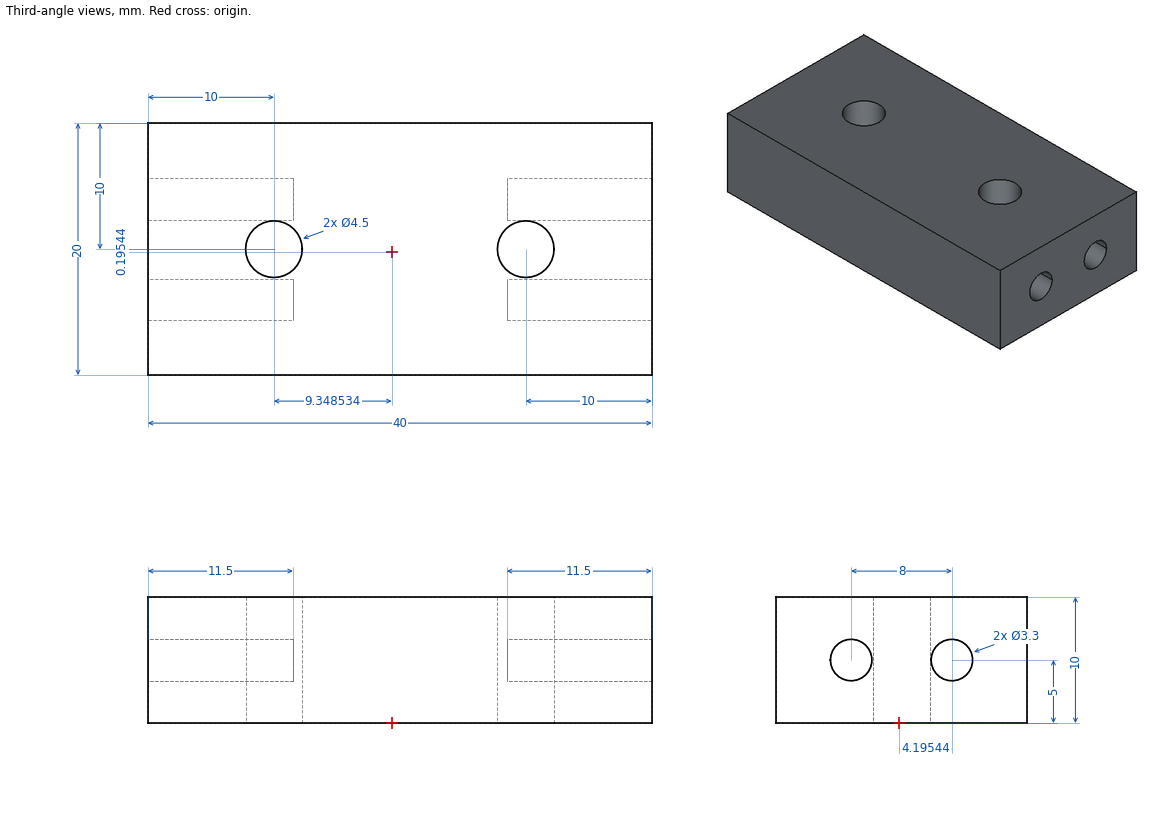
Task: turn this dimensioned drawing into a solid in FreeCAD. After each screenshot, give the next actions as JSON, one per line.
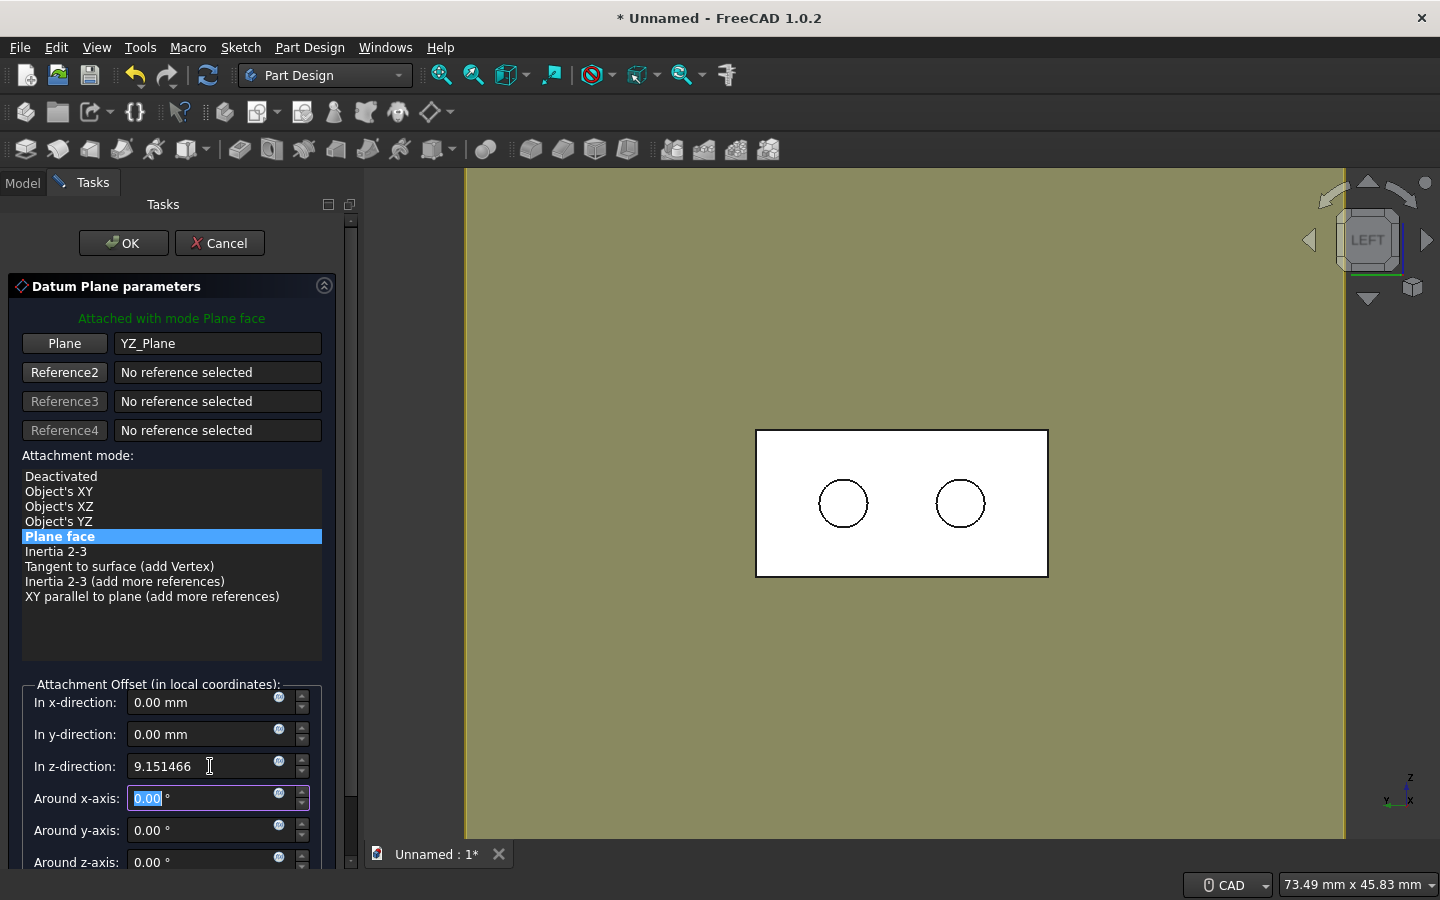
{"action": "left_click", "coordinate": [124, 243]}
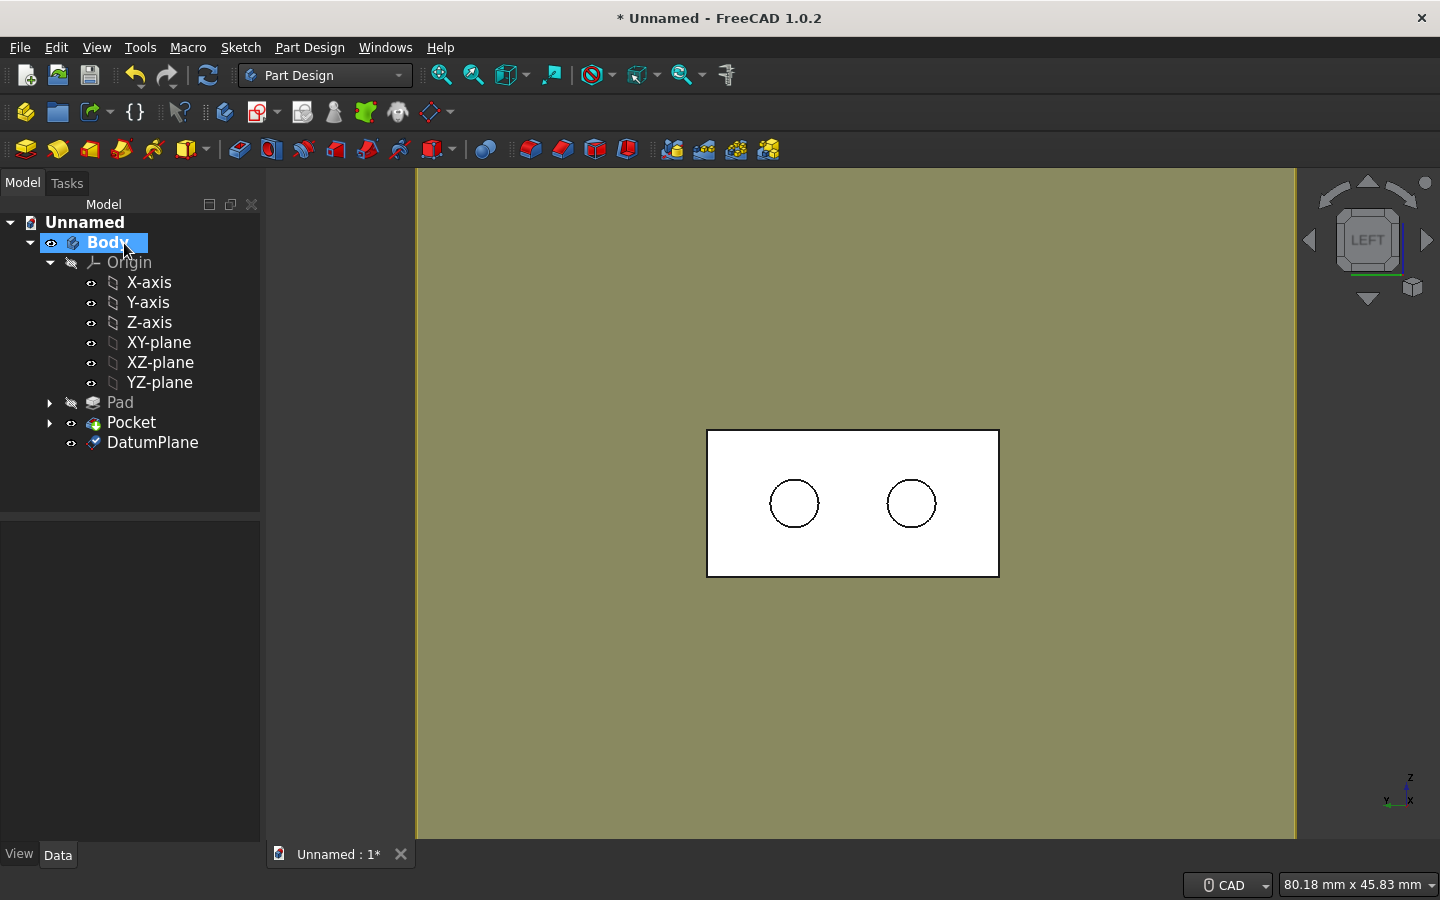
{"action": "left_click", "coordinate": [116, 443]}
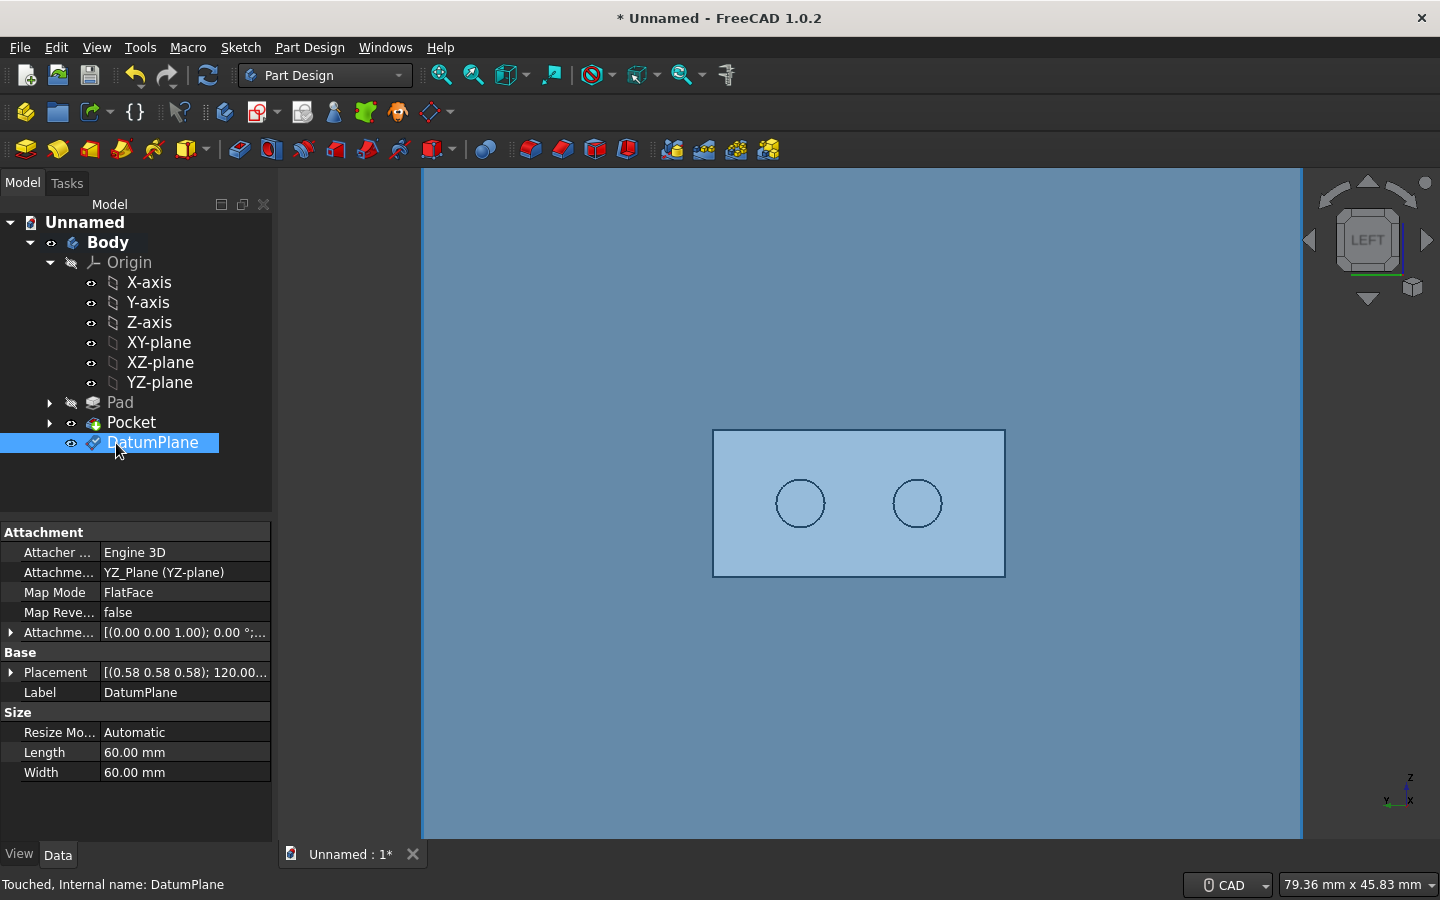
{"action": "left_click", "coordinate": [258, 112]}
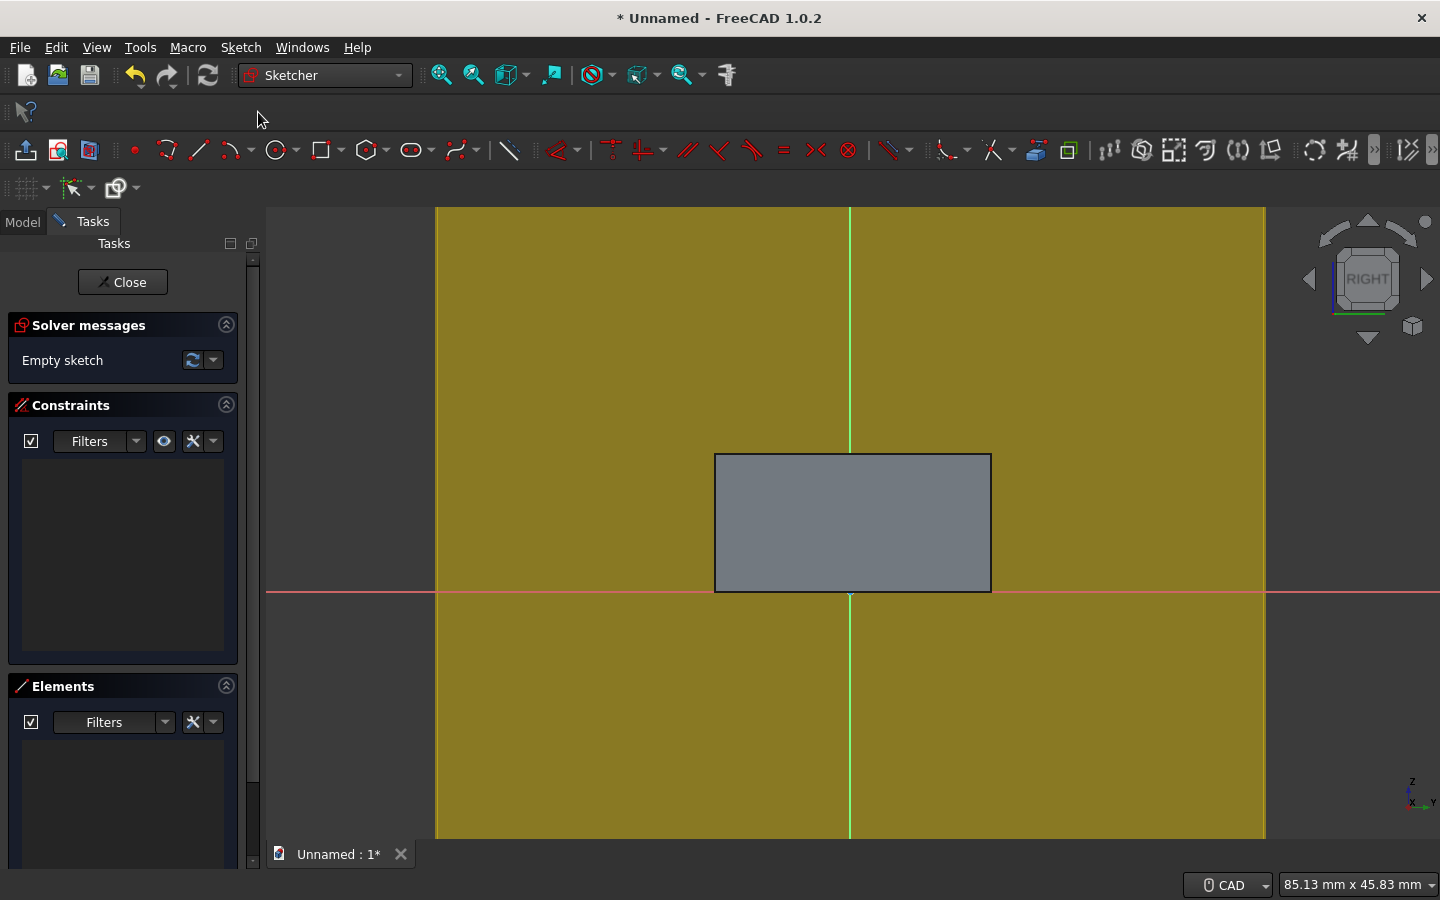
{"action": "key", "text": "q s"}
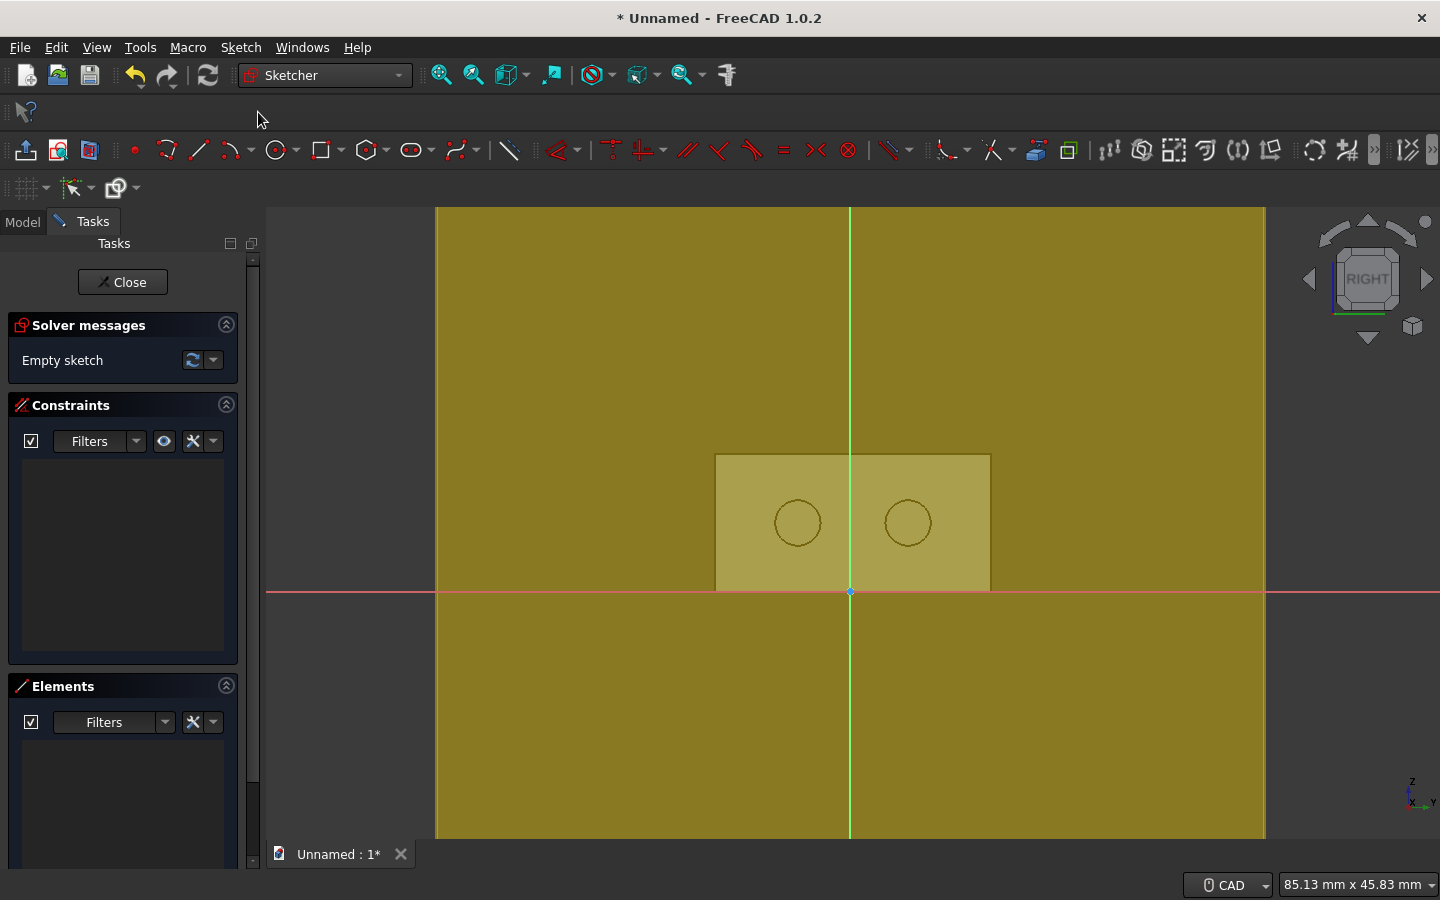
{"action": "scroll", "coordinate": [875, 554], "scroll_direction": "up", "scroll_amount": 7}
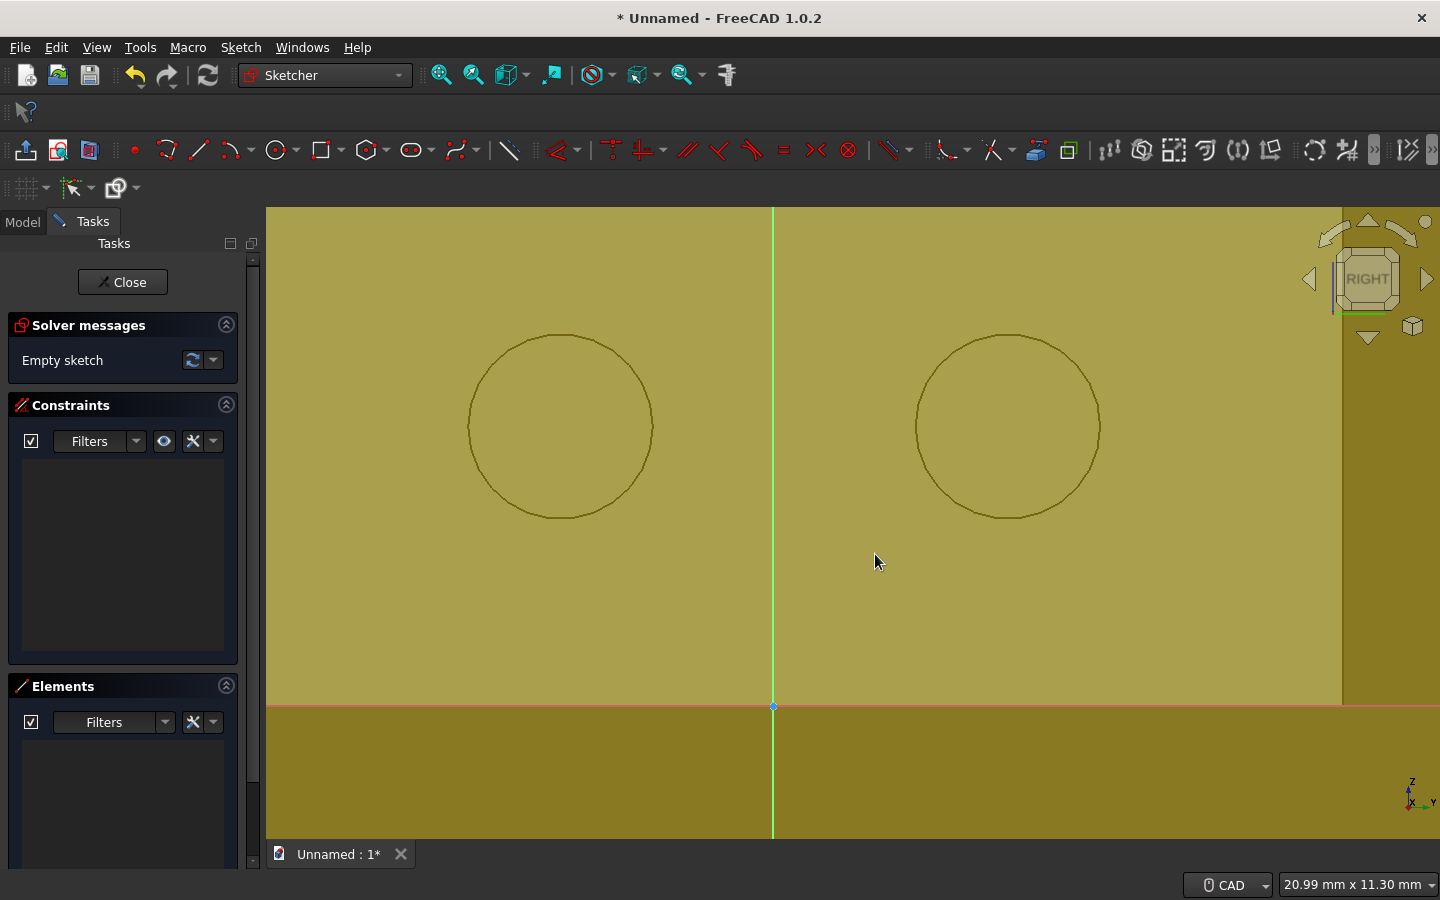
{"action": "left_click", "coordinate": [276, 150]}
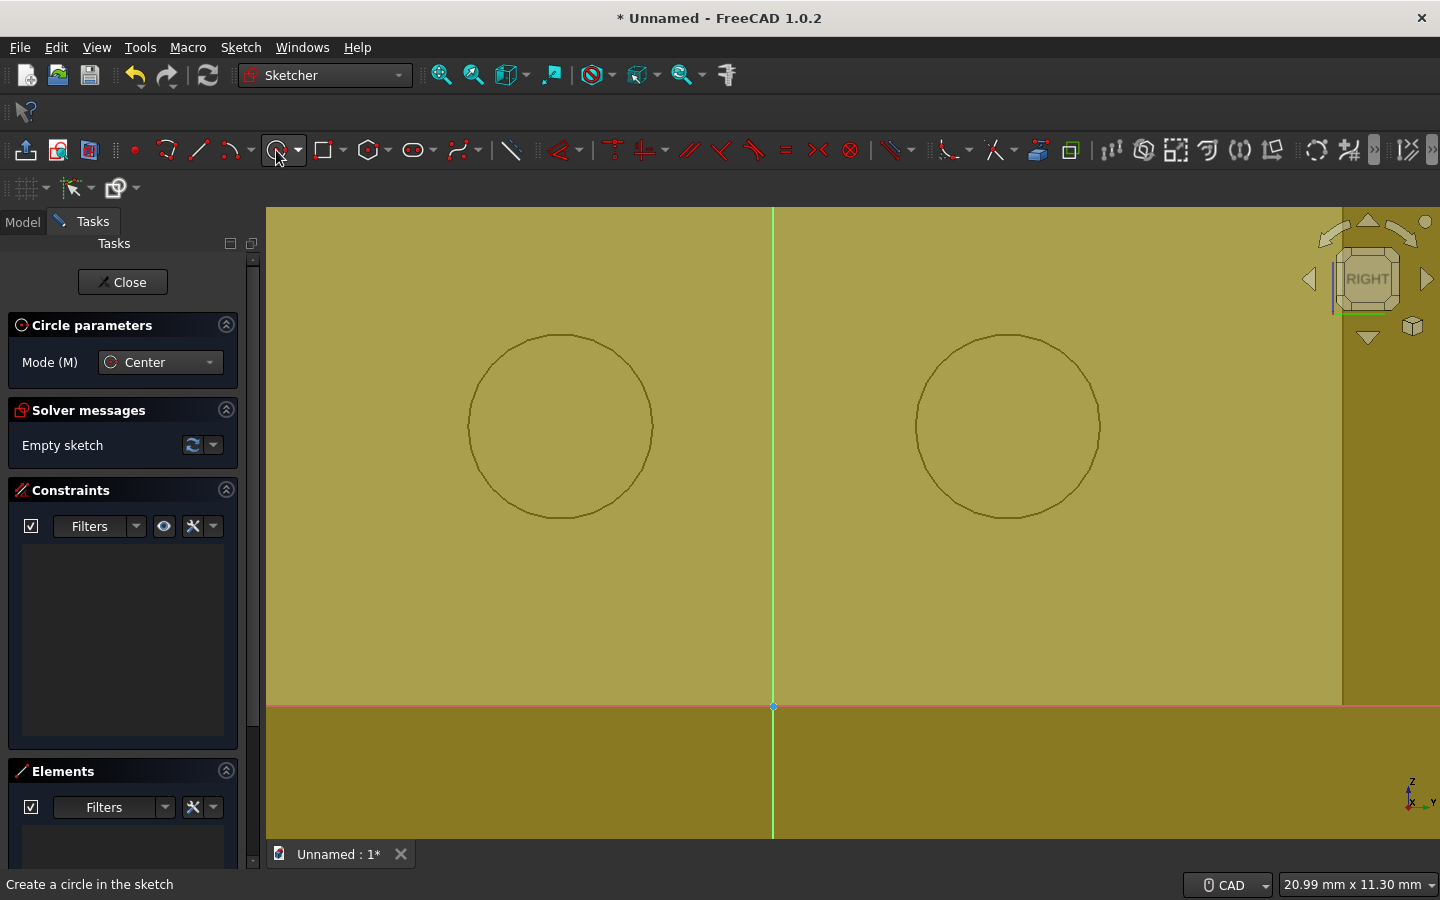
{"action": "left_click", "coordinate": [1008, 427]}
{"action": "left_click", "coordinate": [1073, 361]}